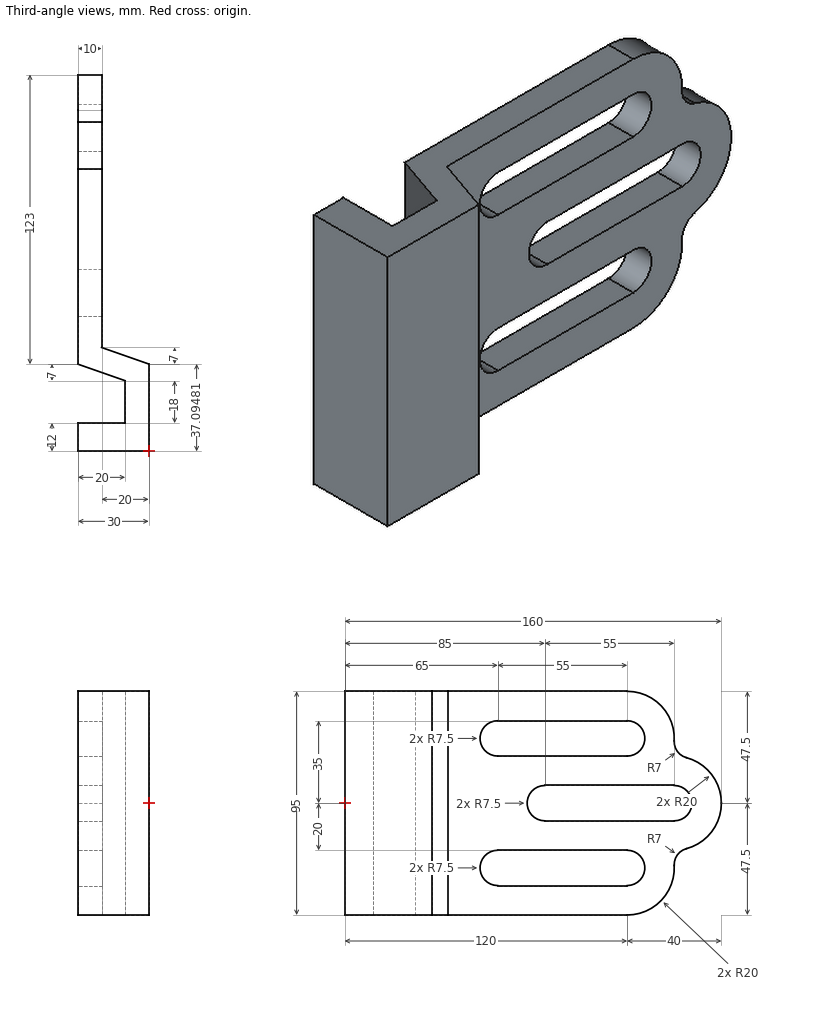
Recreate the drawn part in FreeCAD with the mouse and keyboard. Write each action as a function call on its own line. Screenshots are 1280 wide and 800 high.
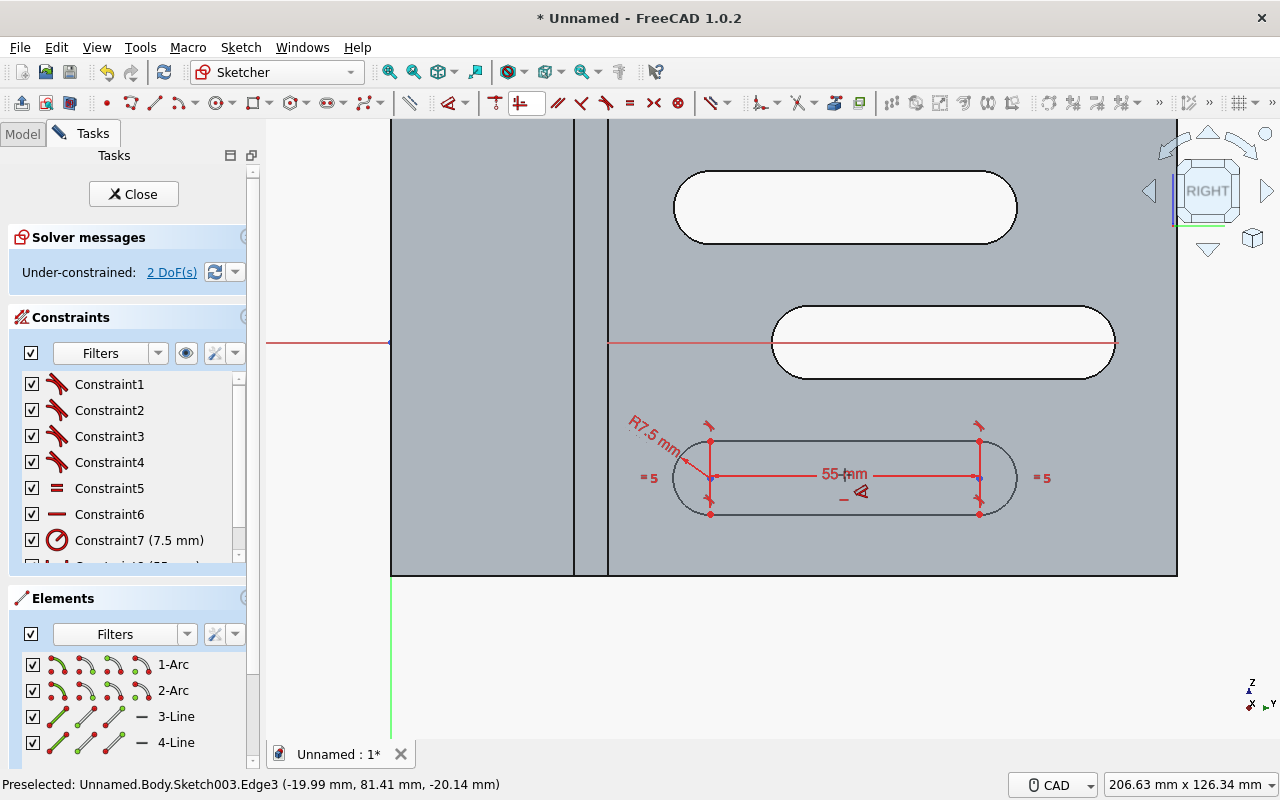
click(710, 441)
click(551, 309)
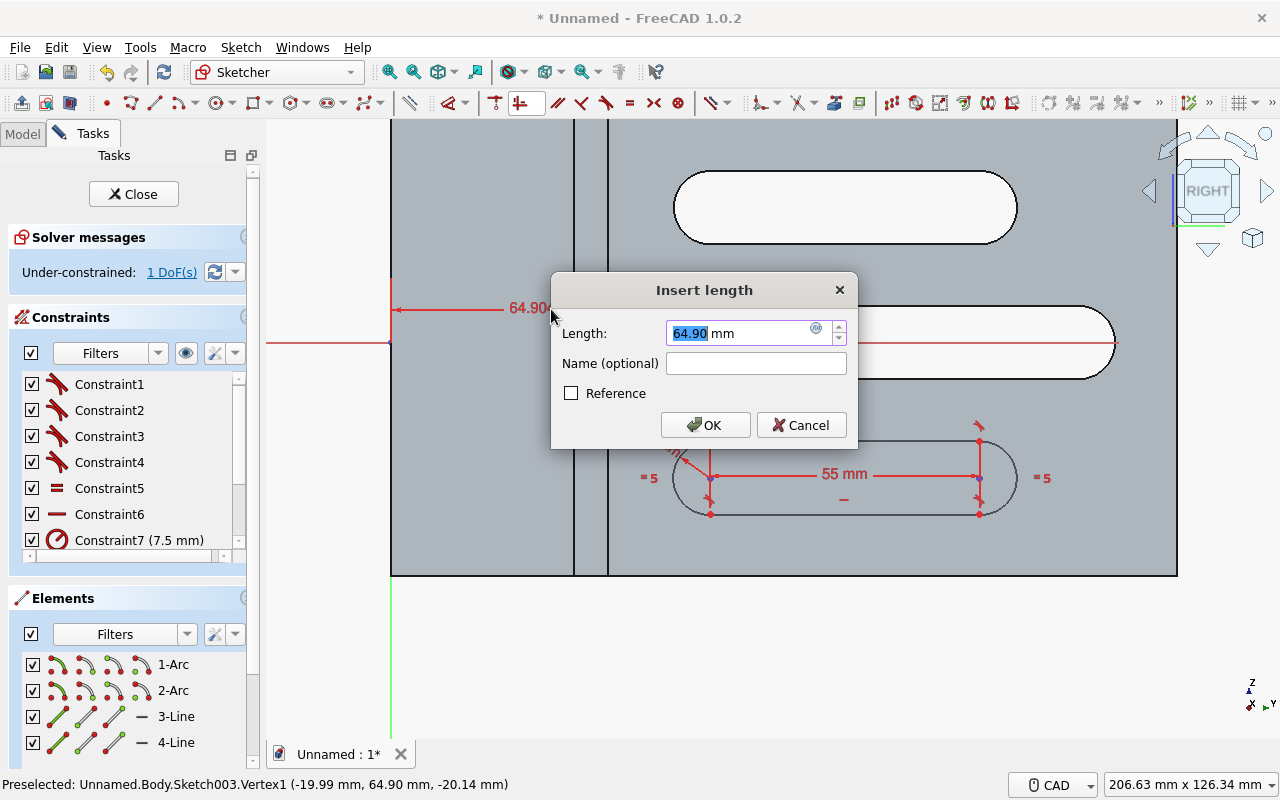
text(65)
key(Return)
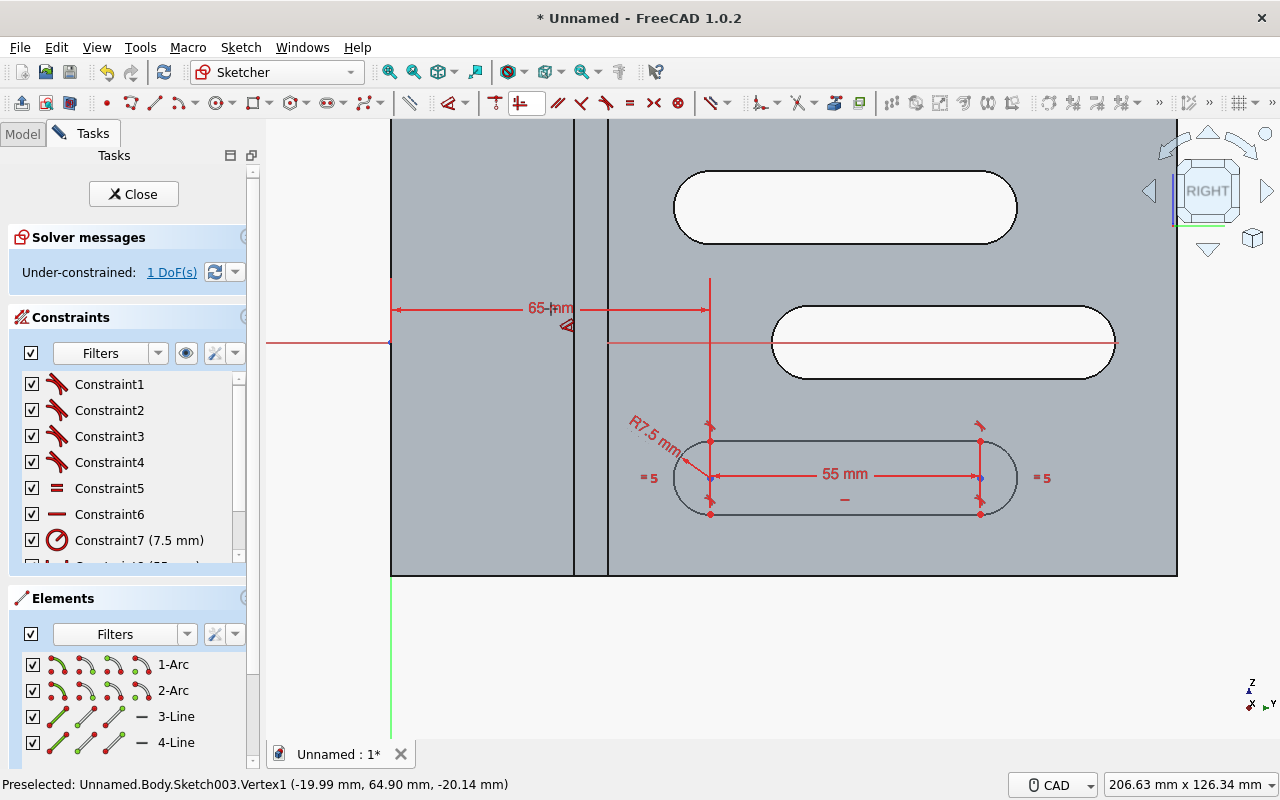
click(710, 441)
click(357, 392)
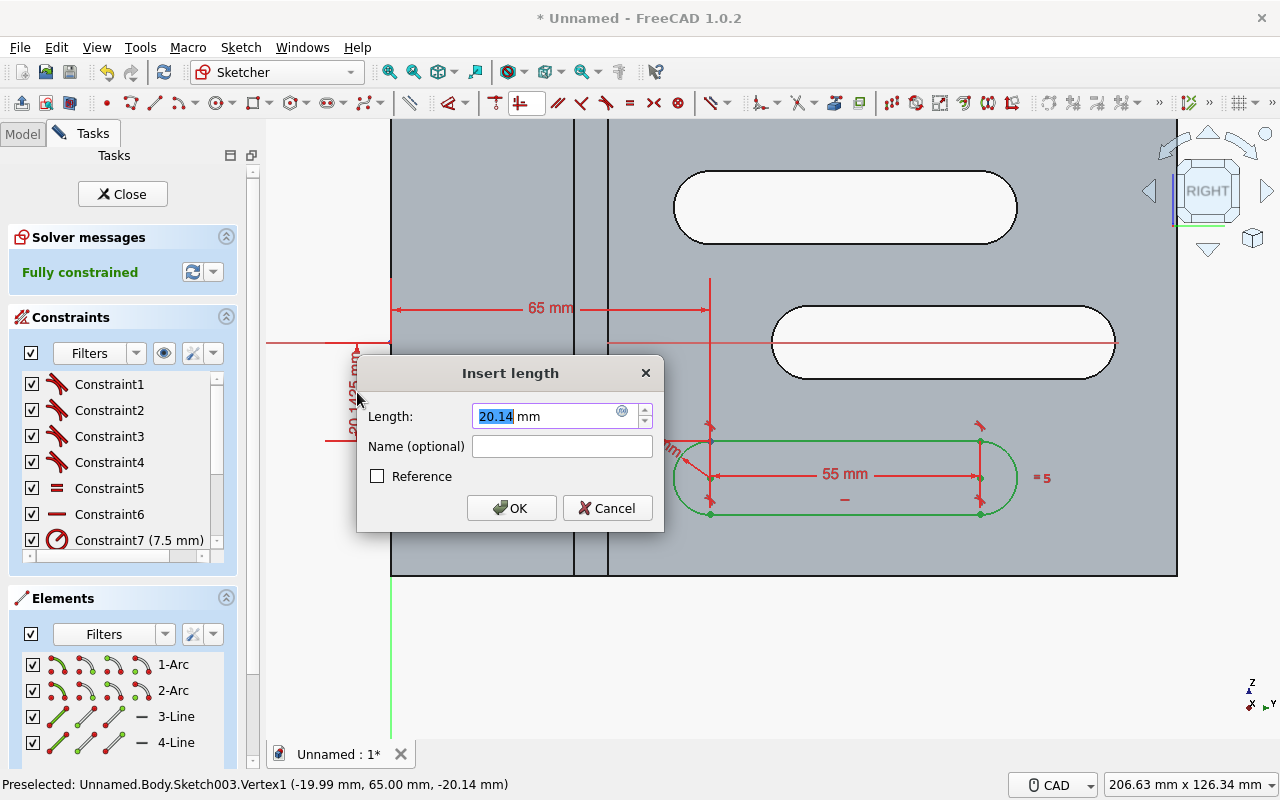
text(20)
key(Return)
key(Escape)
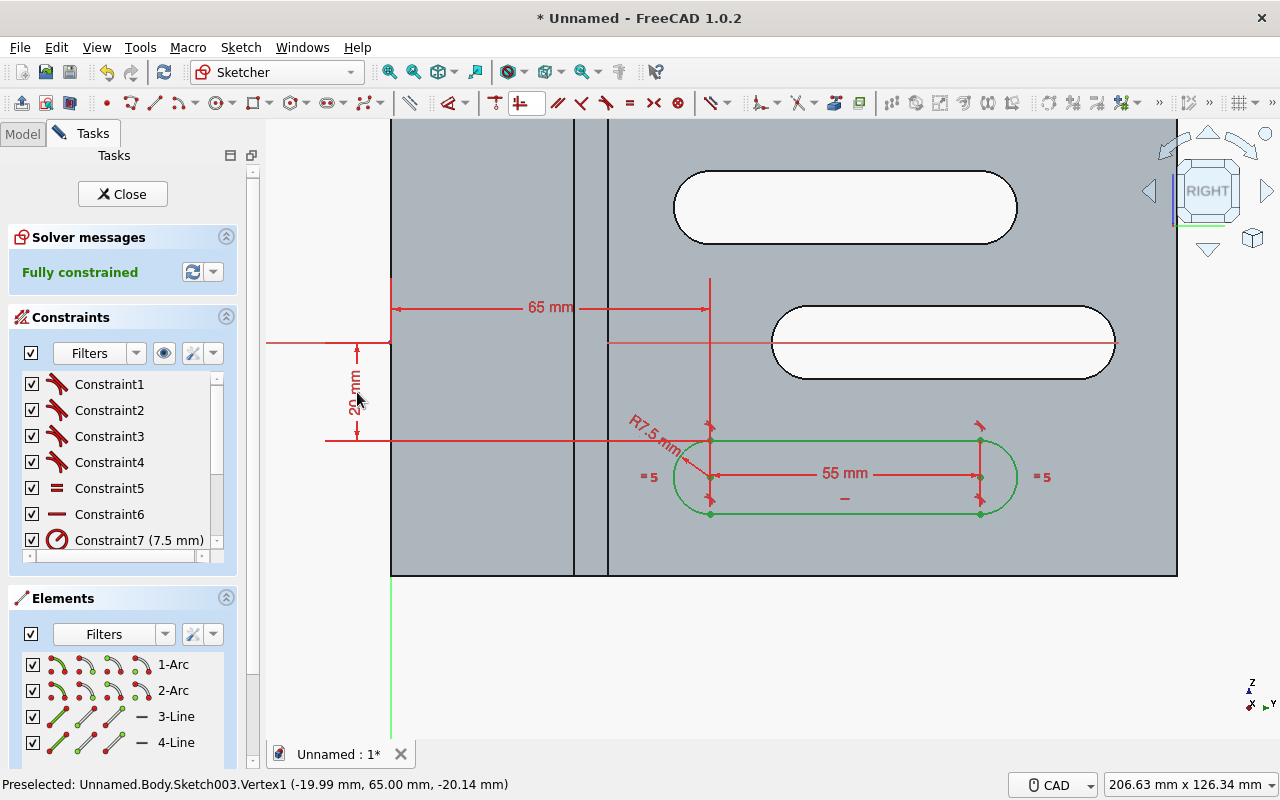
click(123, 194)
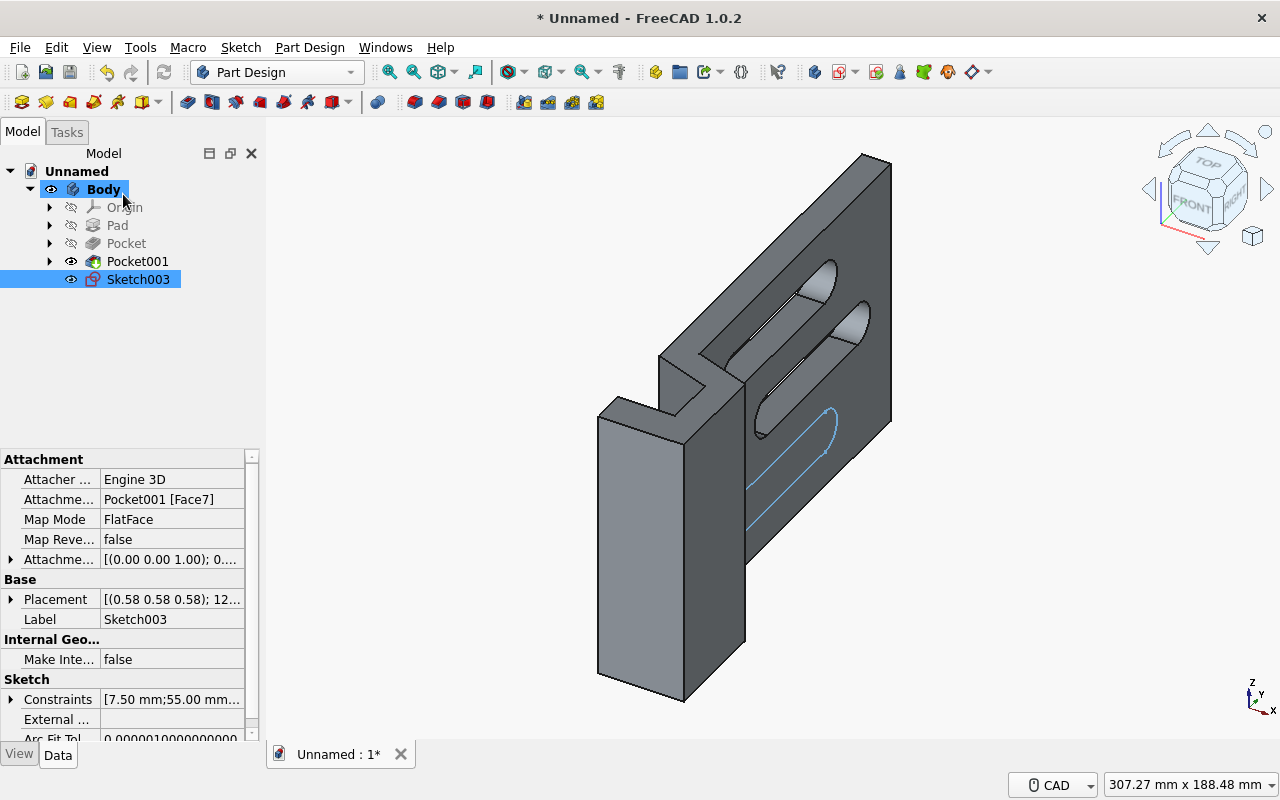
click(188, 102)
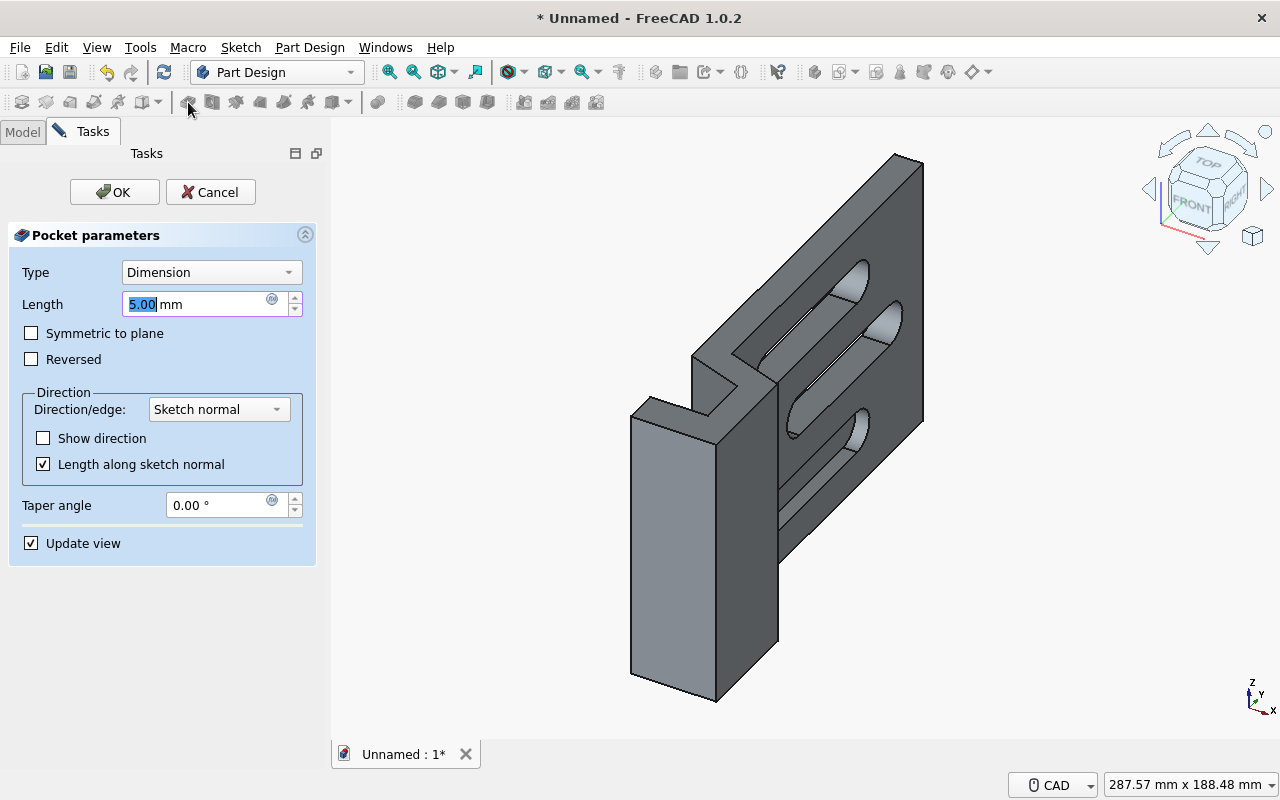
click(212, 272)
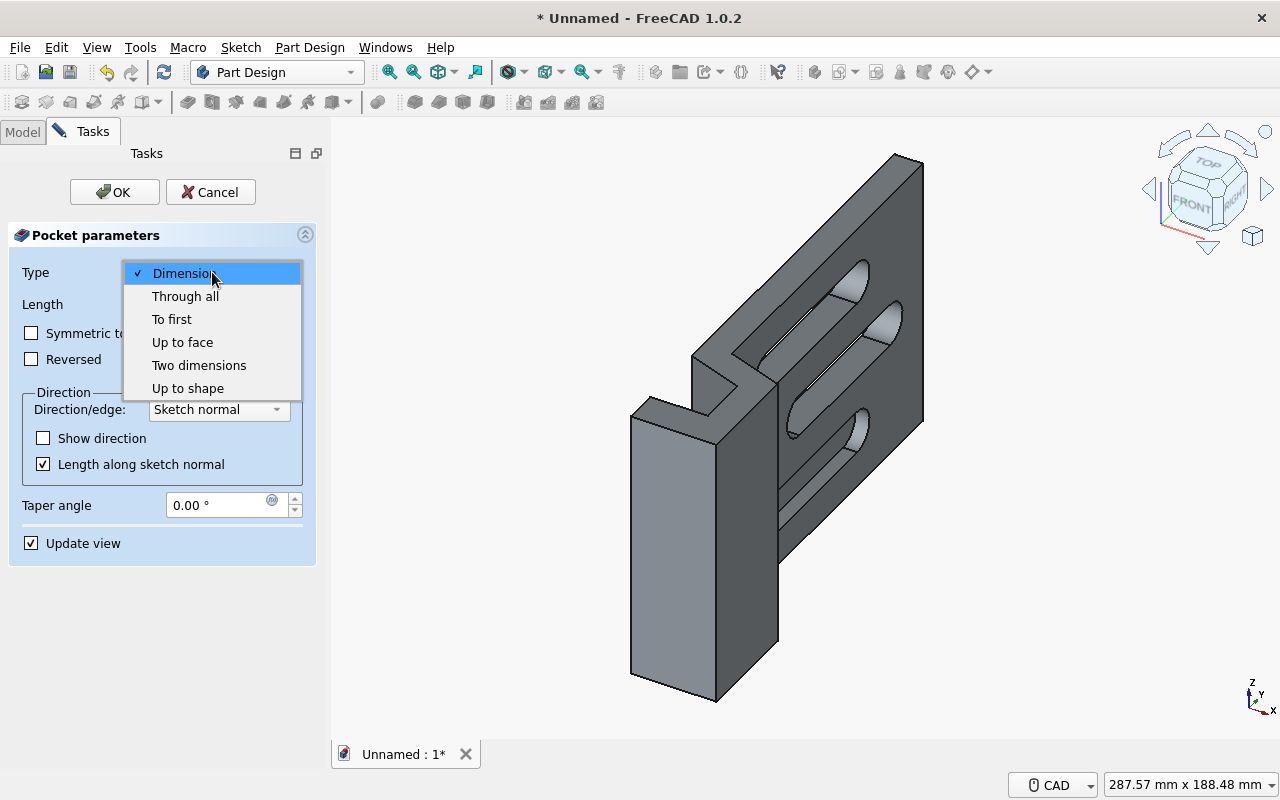
click(212, 320)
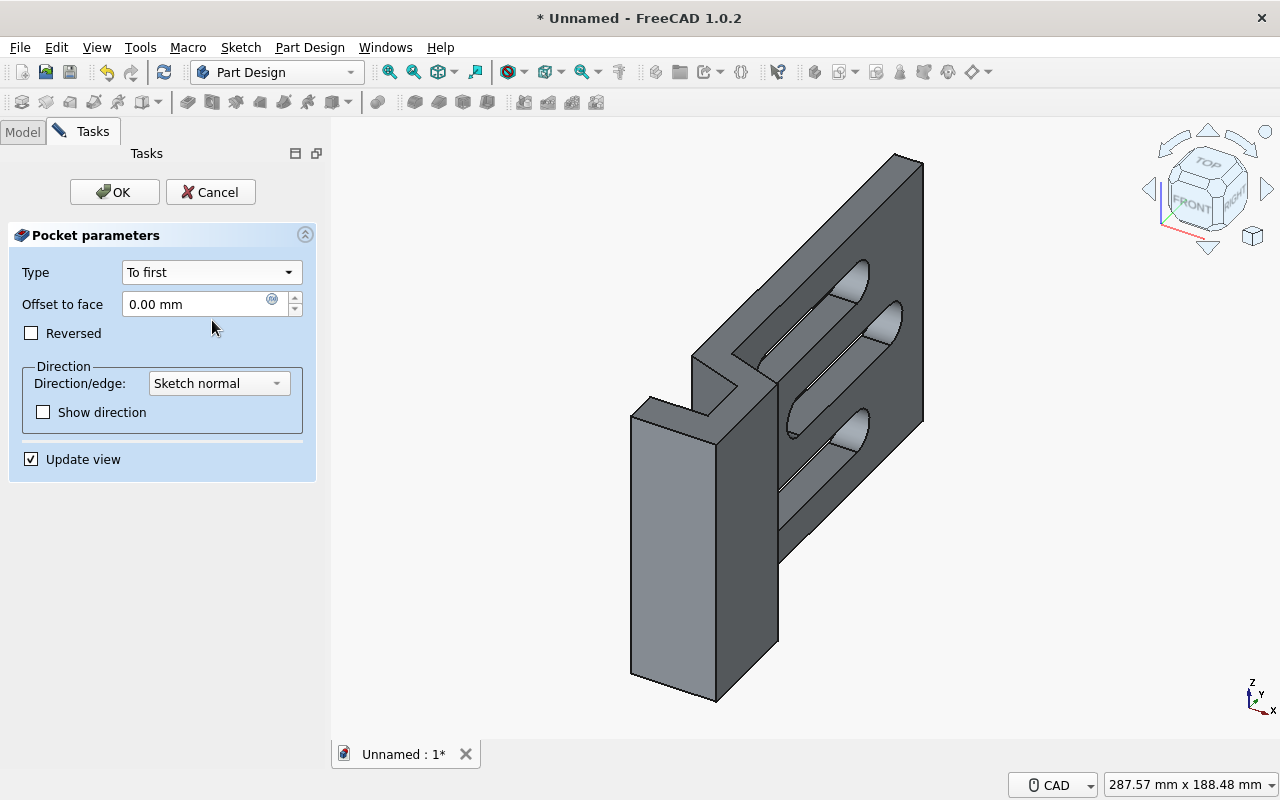
click(115, 192)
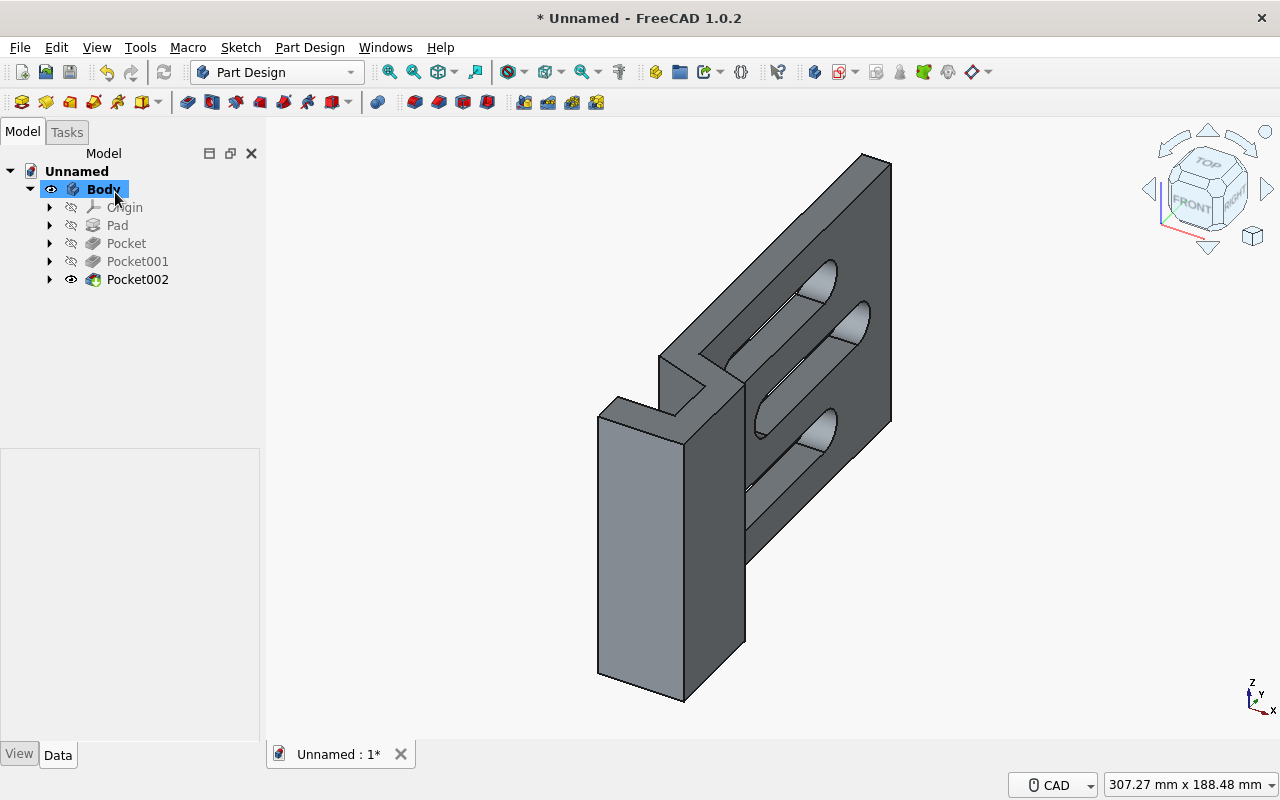
click(877, 231)